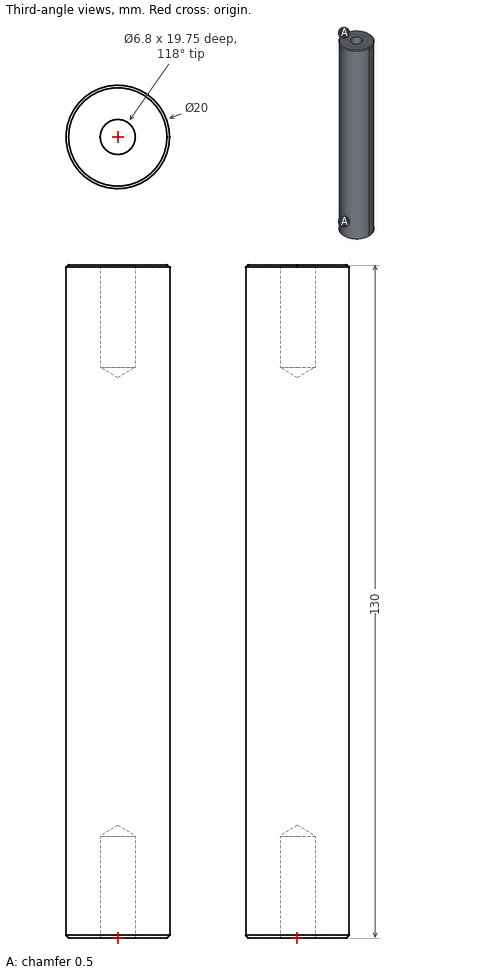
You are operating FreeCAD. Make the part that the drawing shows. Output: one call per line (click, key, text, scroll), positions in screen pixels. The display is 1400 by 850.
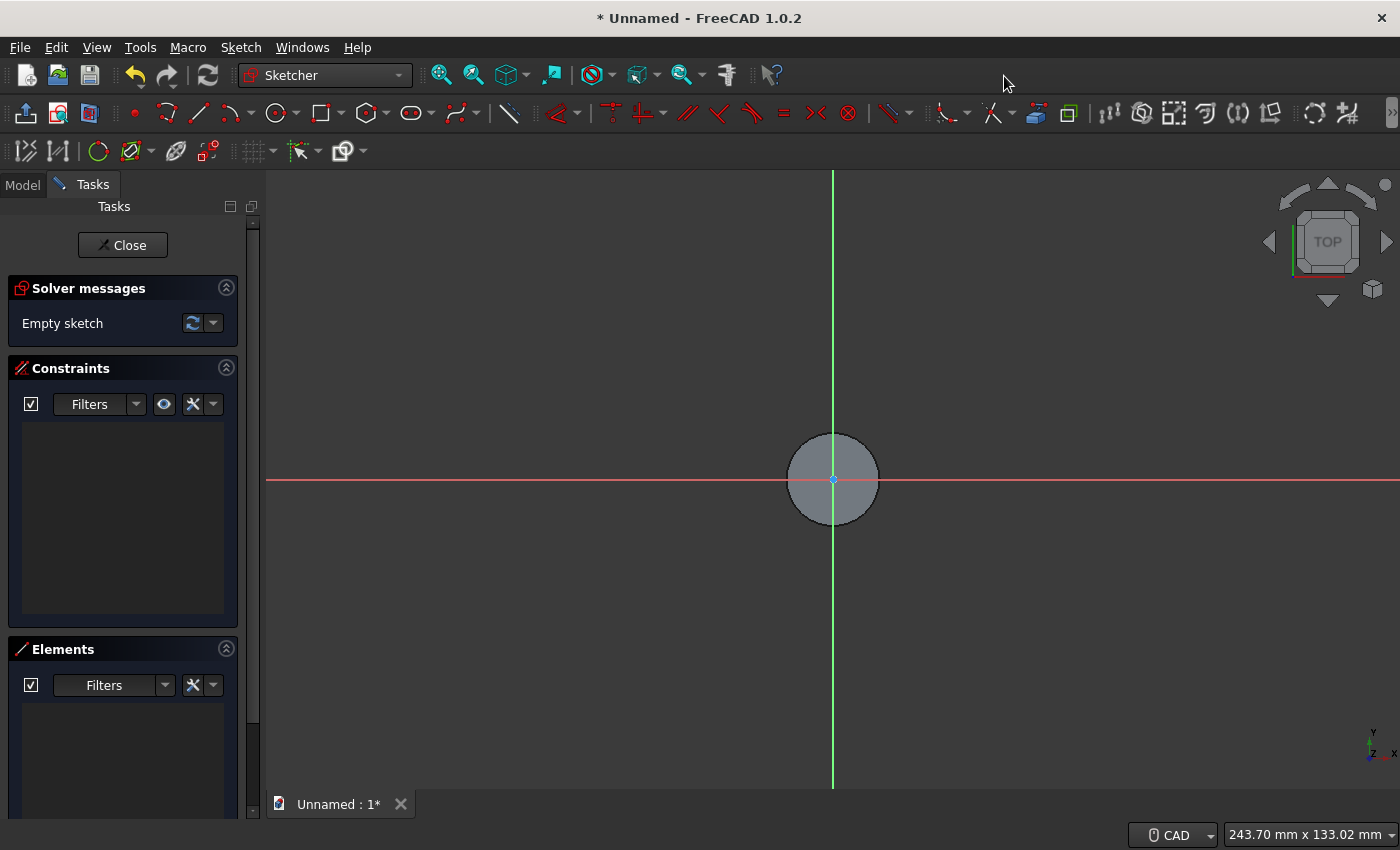
scroll(838, 480, up, 13)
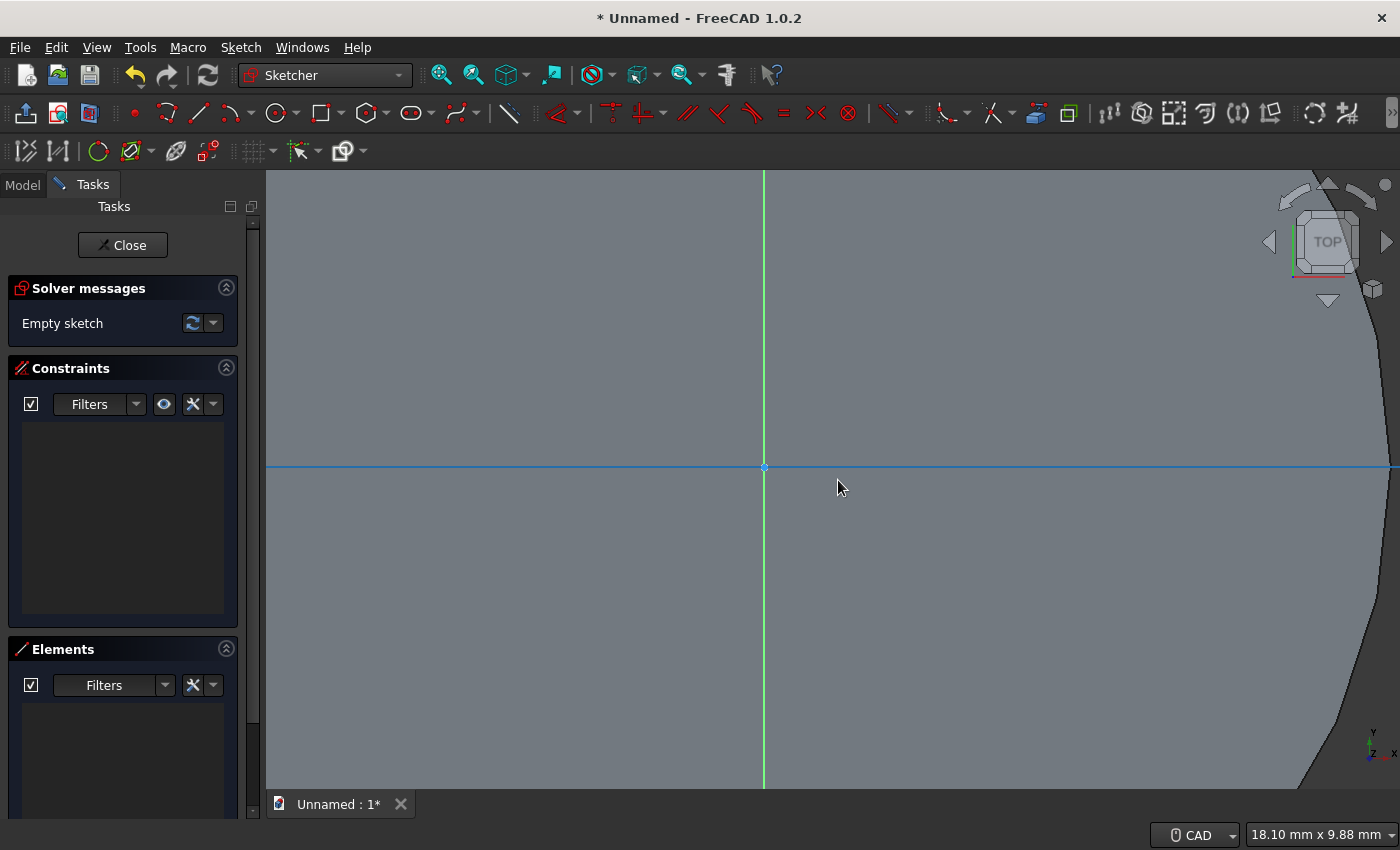
key(g)
key(c)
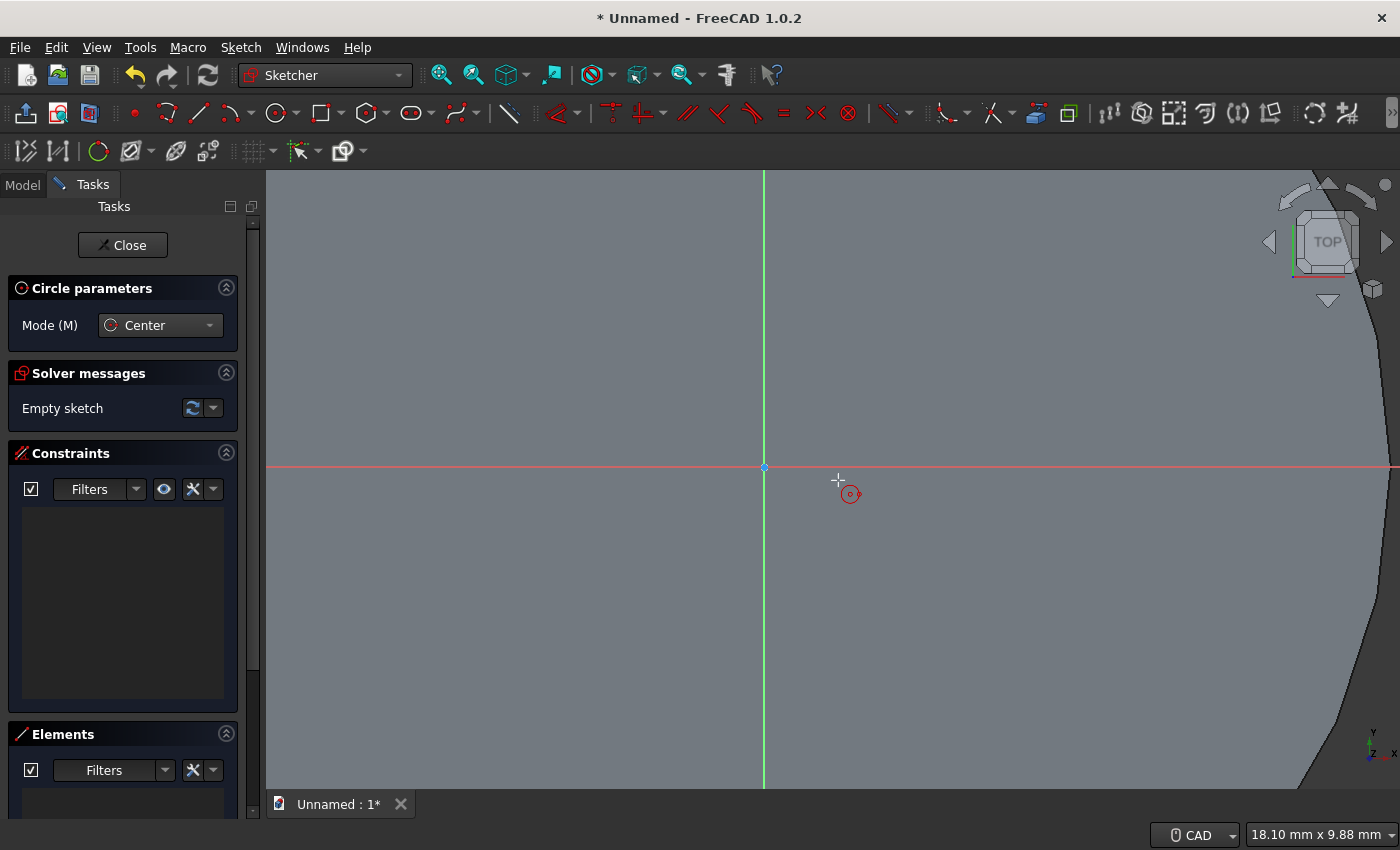
click(764, 467)
click(915, 316)
key(Escape)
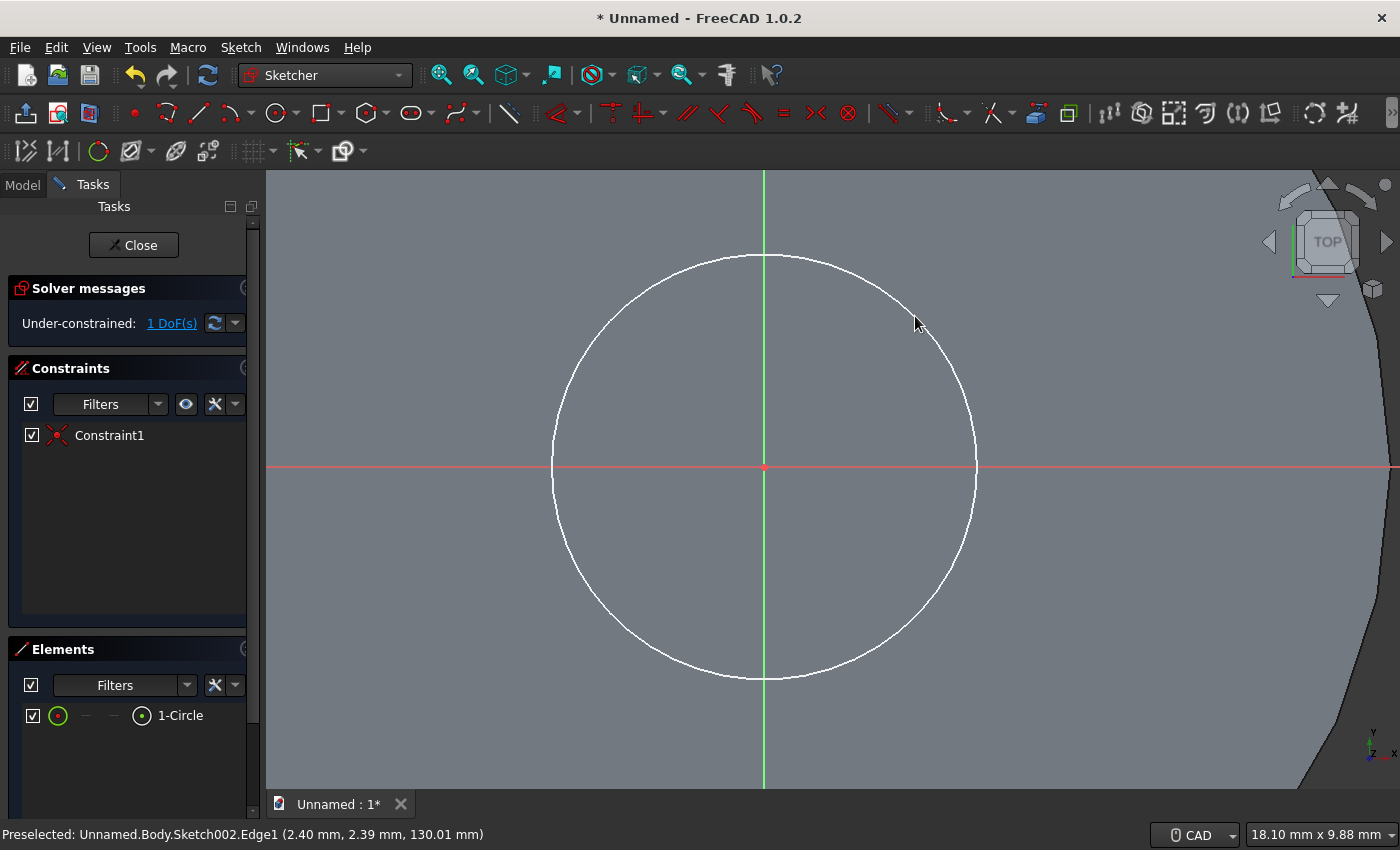
click(556, 114)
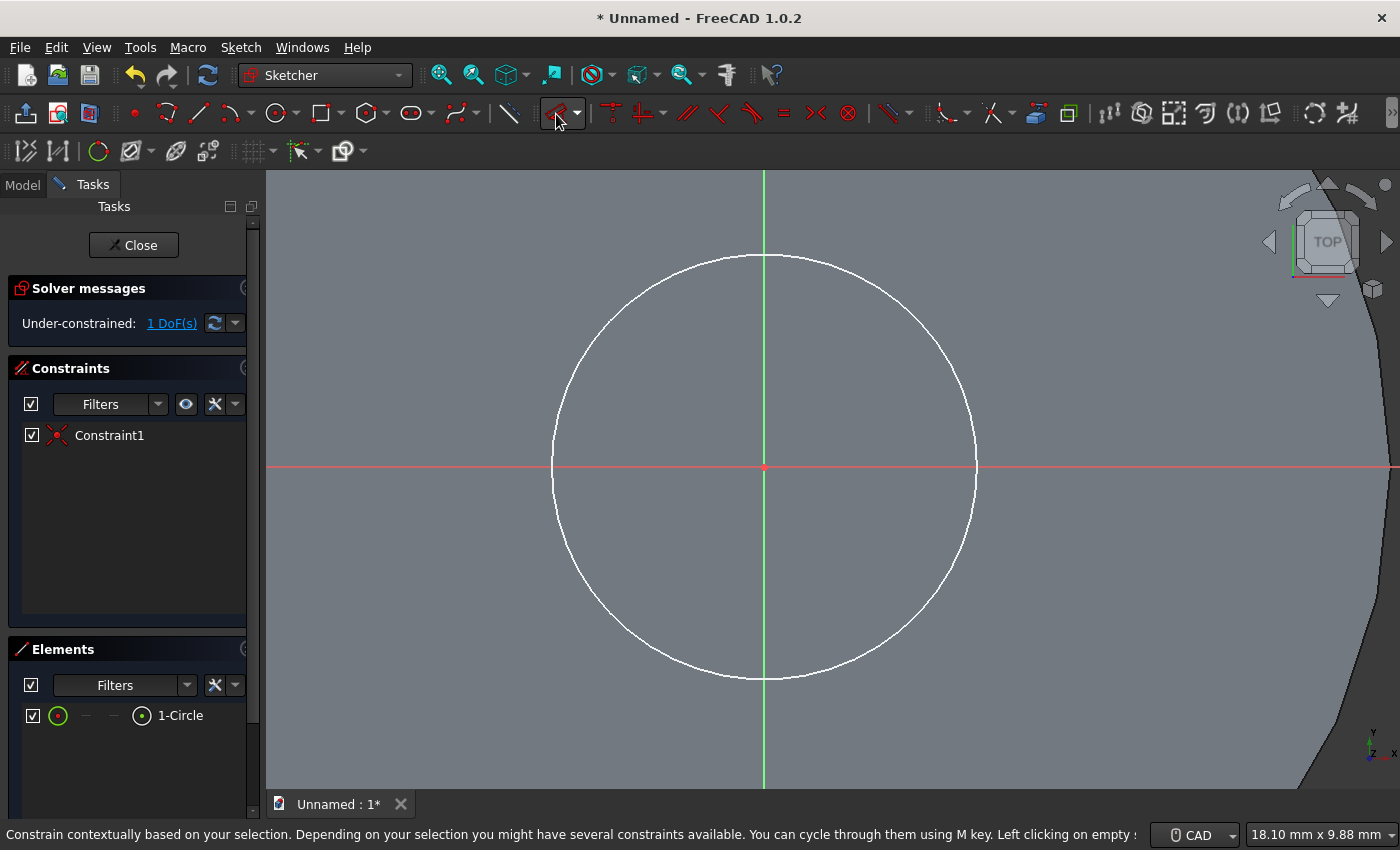
click(914, 316)
click(937, 293)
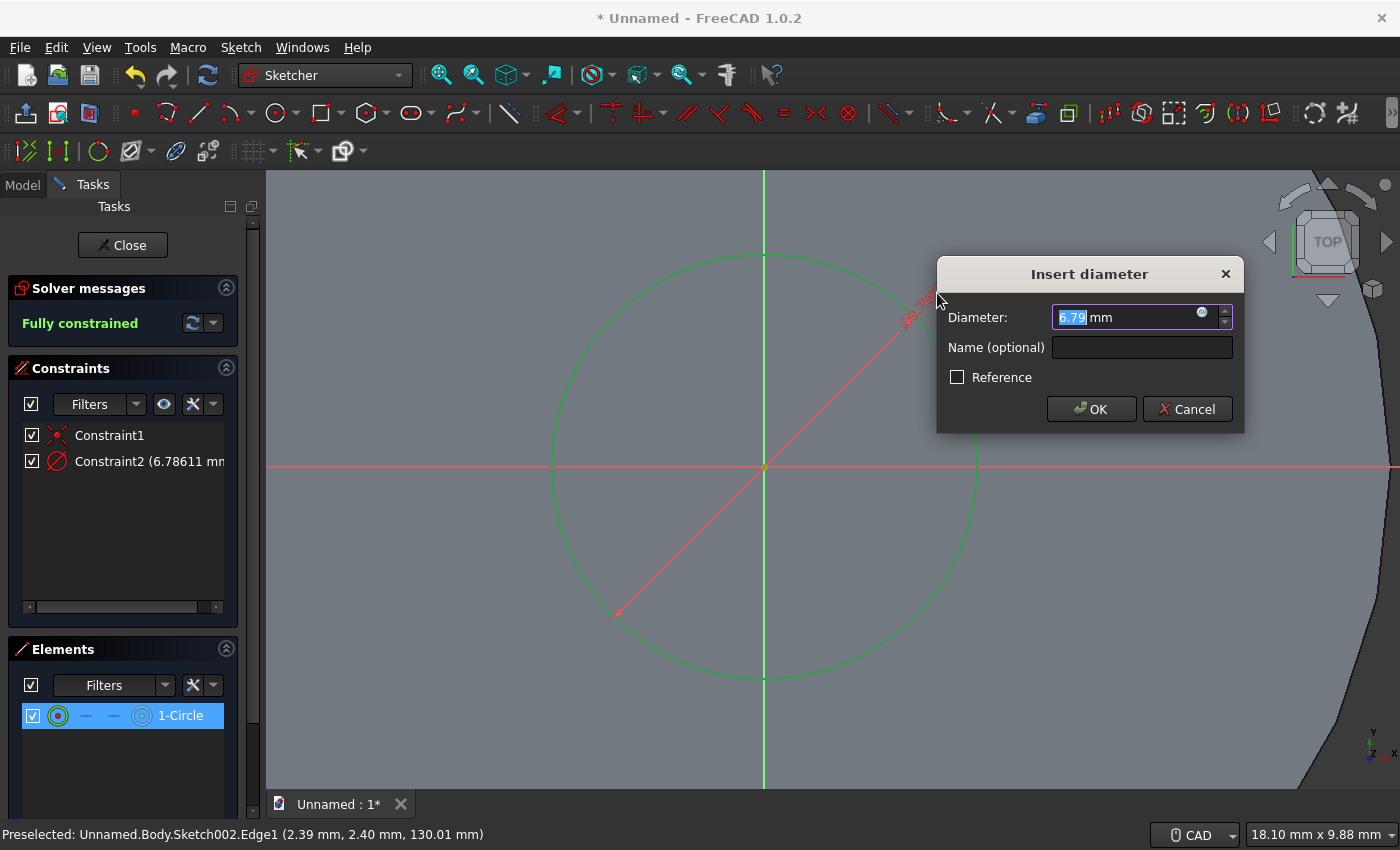
text(6.8)
key(Return)
key(Escape)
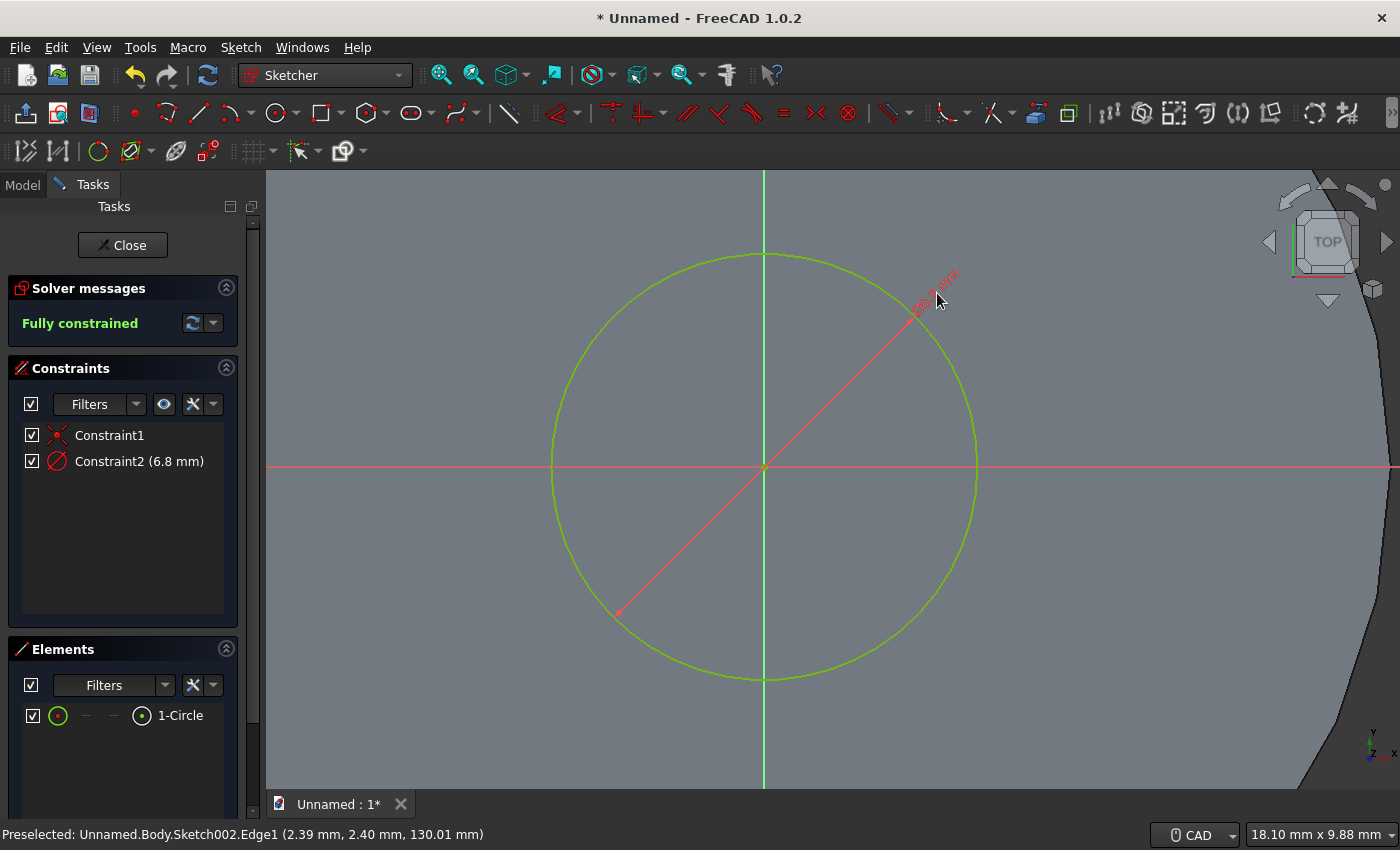
click(123, 245)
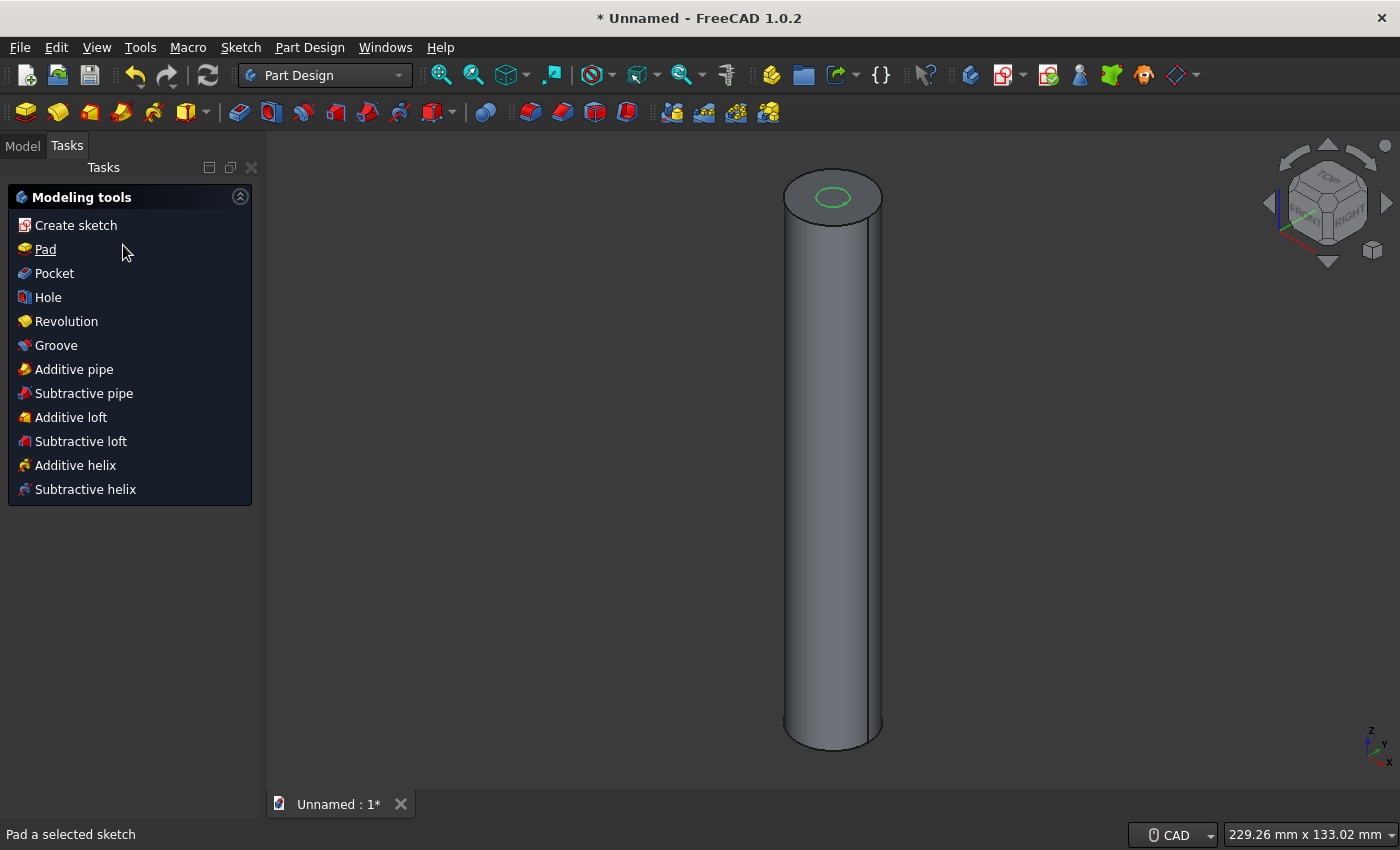
click(272, 112)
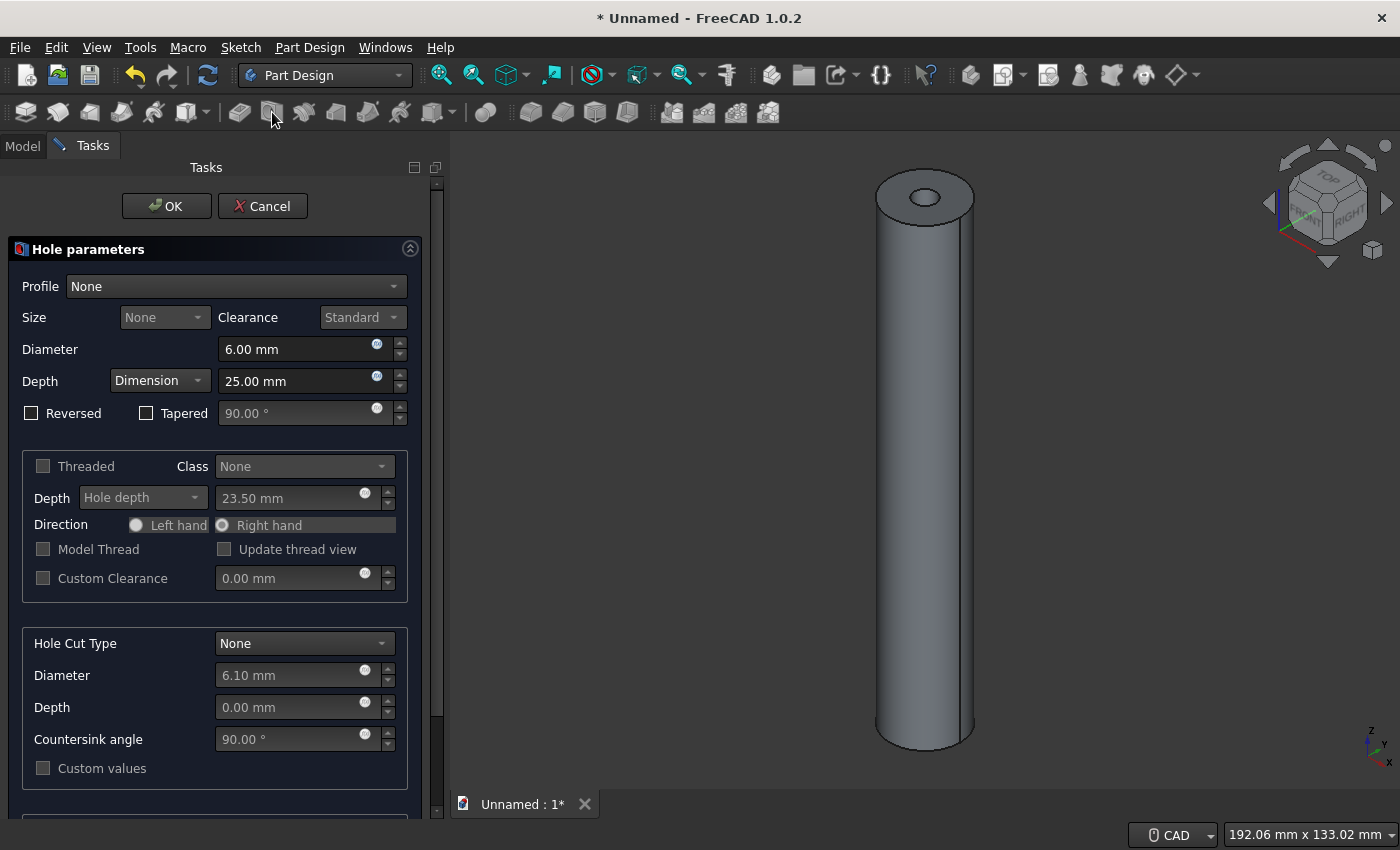
triple_click(305, 349)